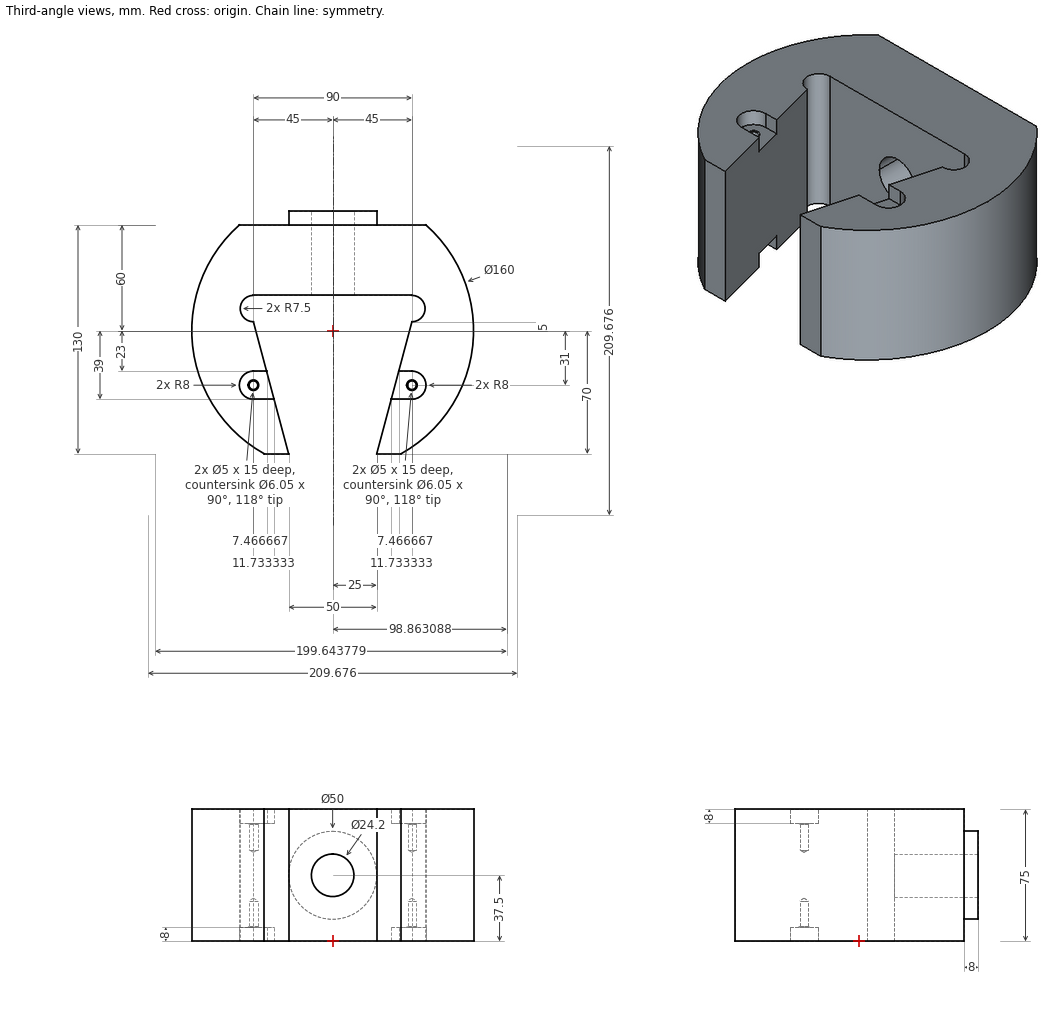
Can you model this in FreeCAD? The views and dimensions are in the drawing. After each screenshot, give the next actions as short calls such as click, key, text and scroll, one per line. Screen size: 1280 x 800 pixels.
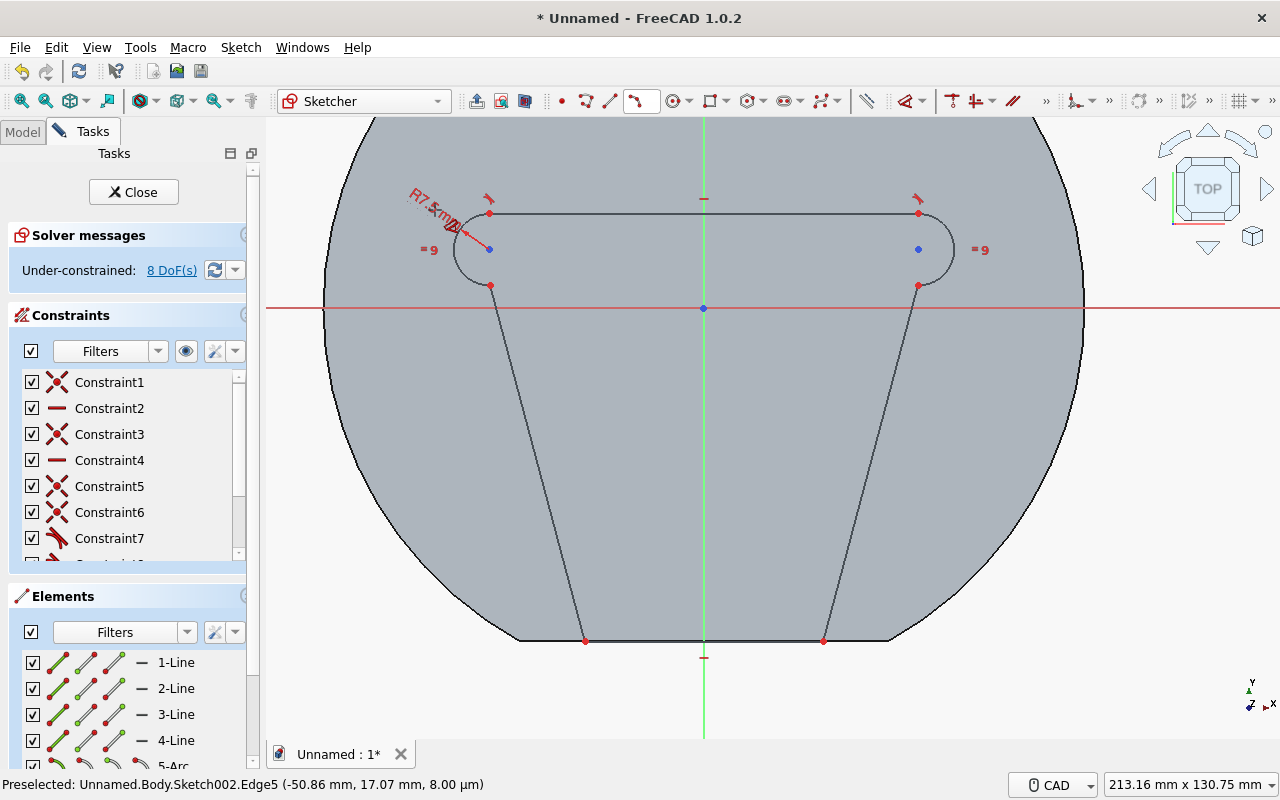
click(752, 642)
click(649, 676)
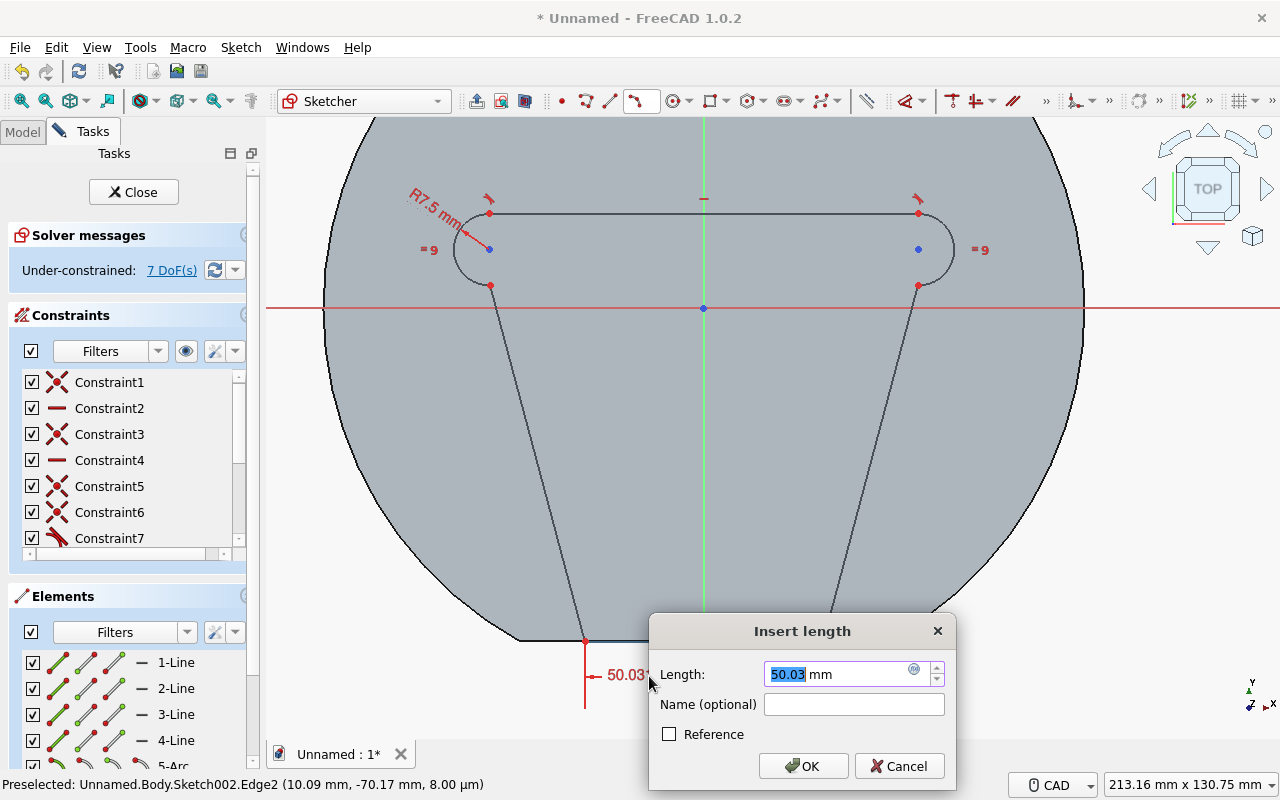
text(50)
key(Return)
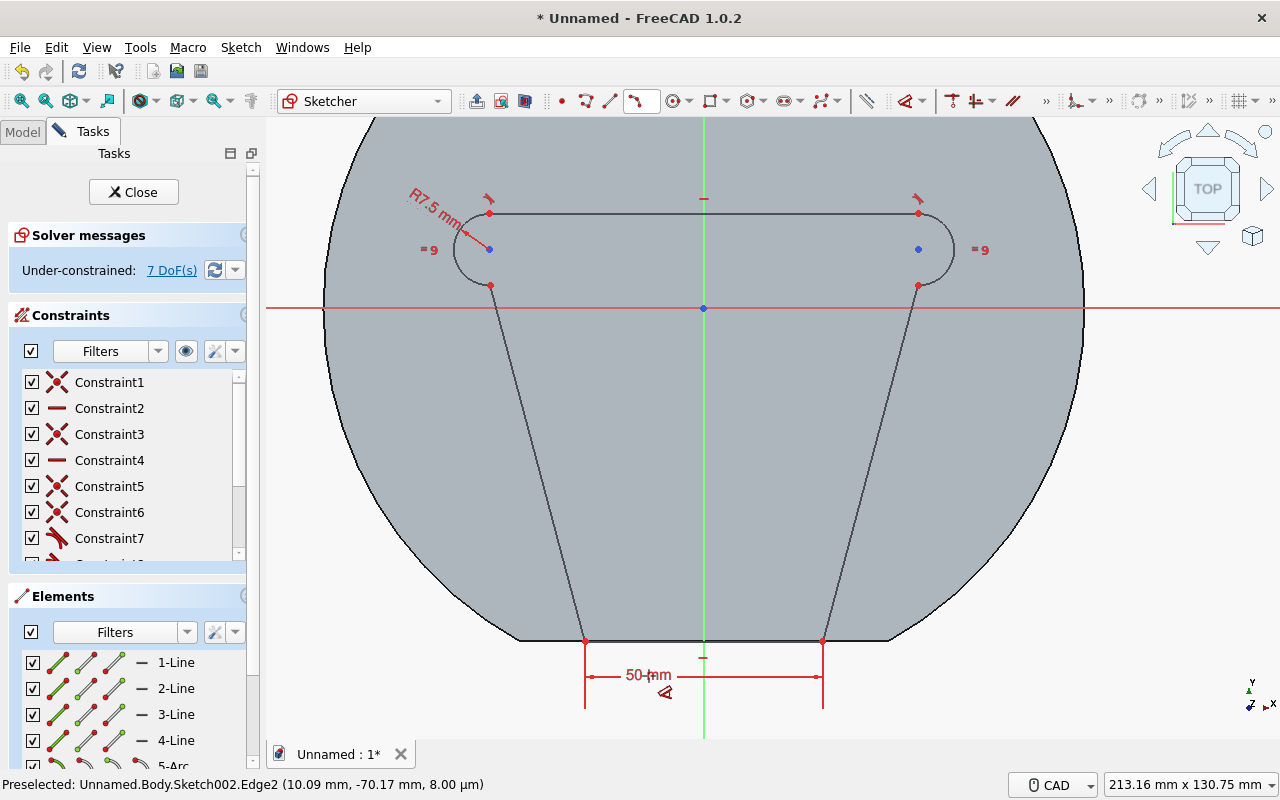
click(618, 214)
click(605, 180)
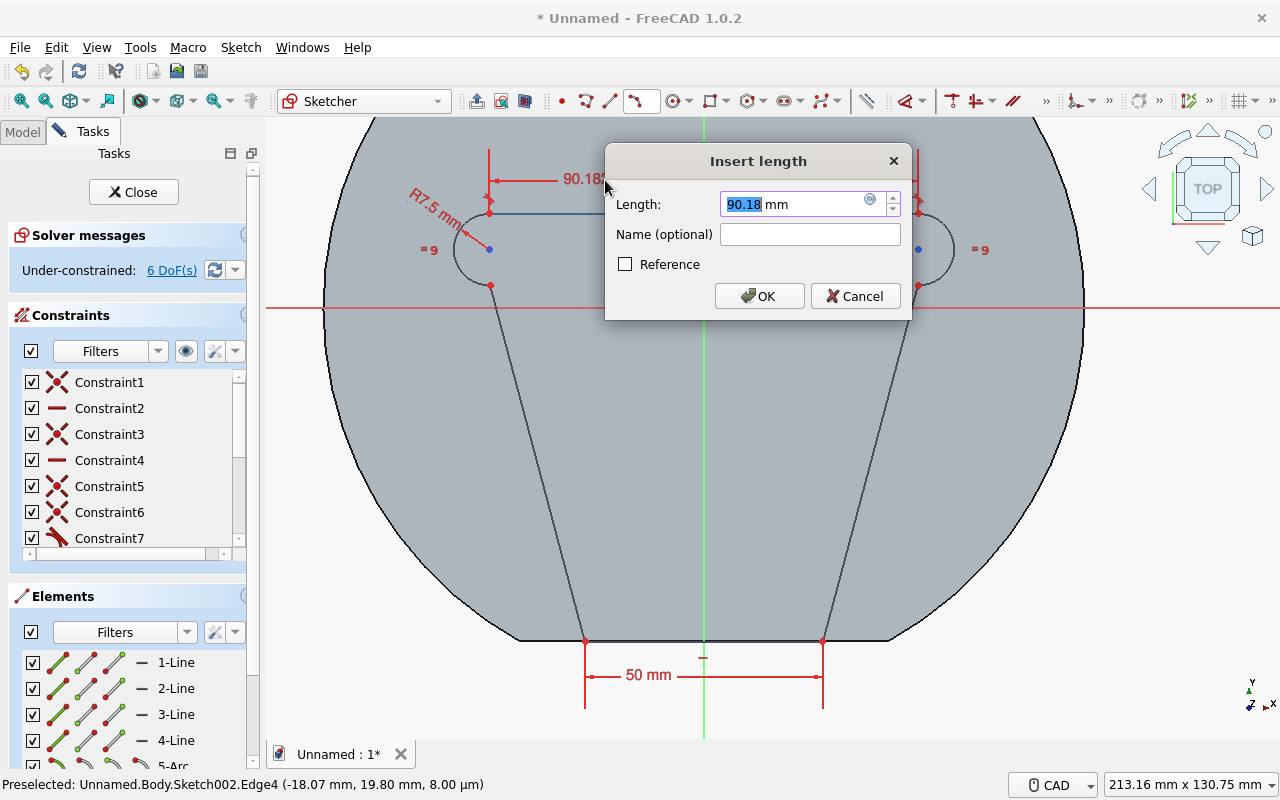
text(90)
key(Return)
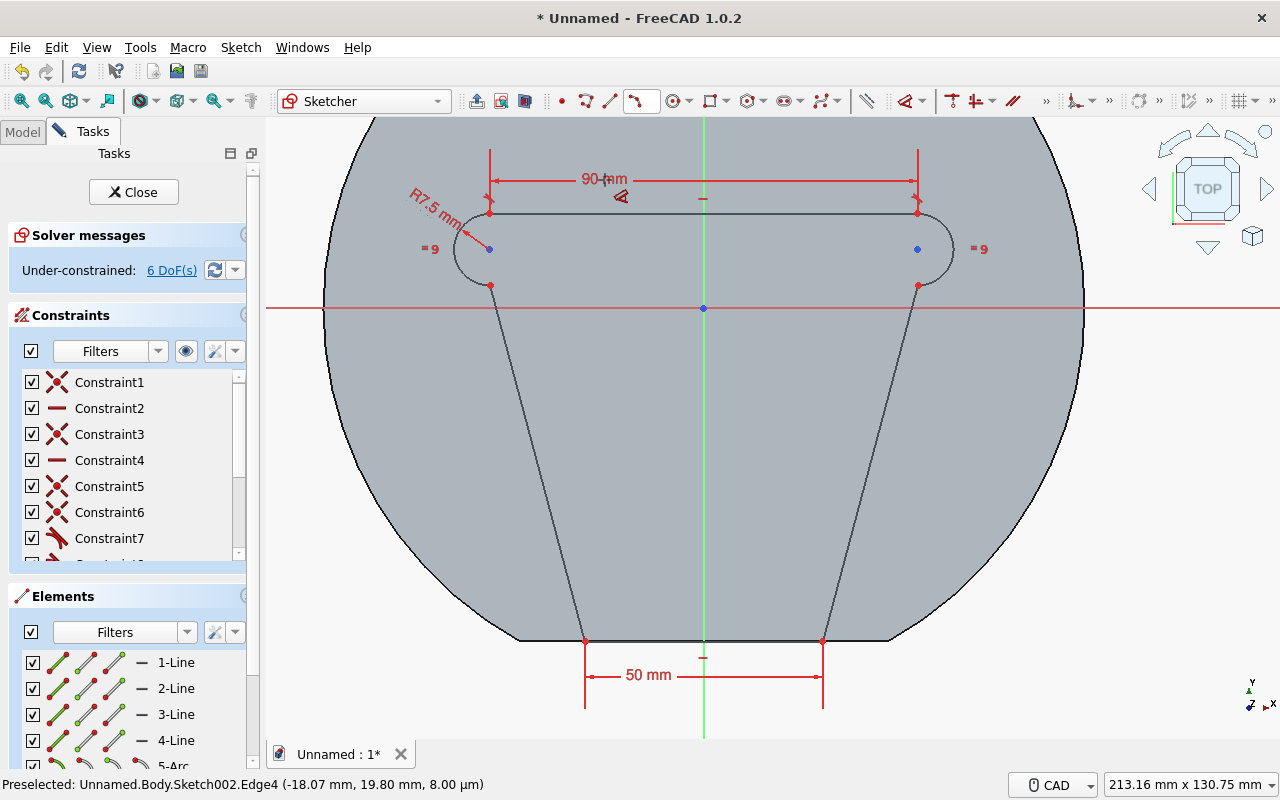
scroll(918, 285, up, 3)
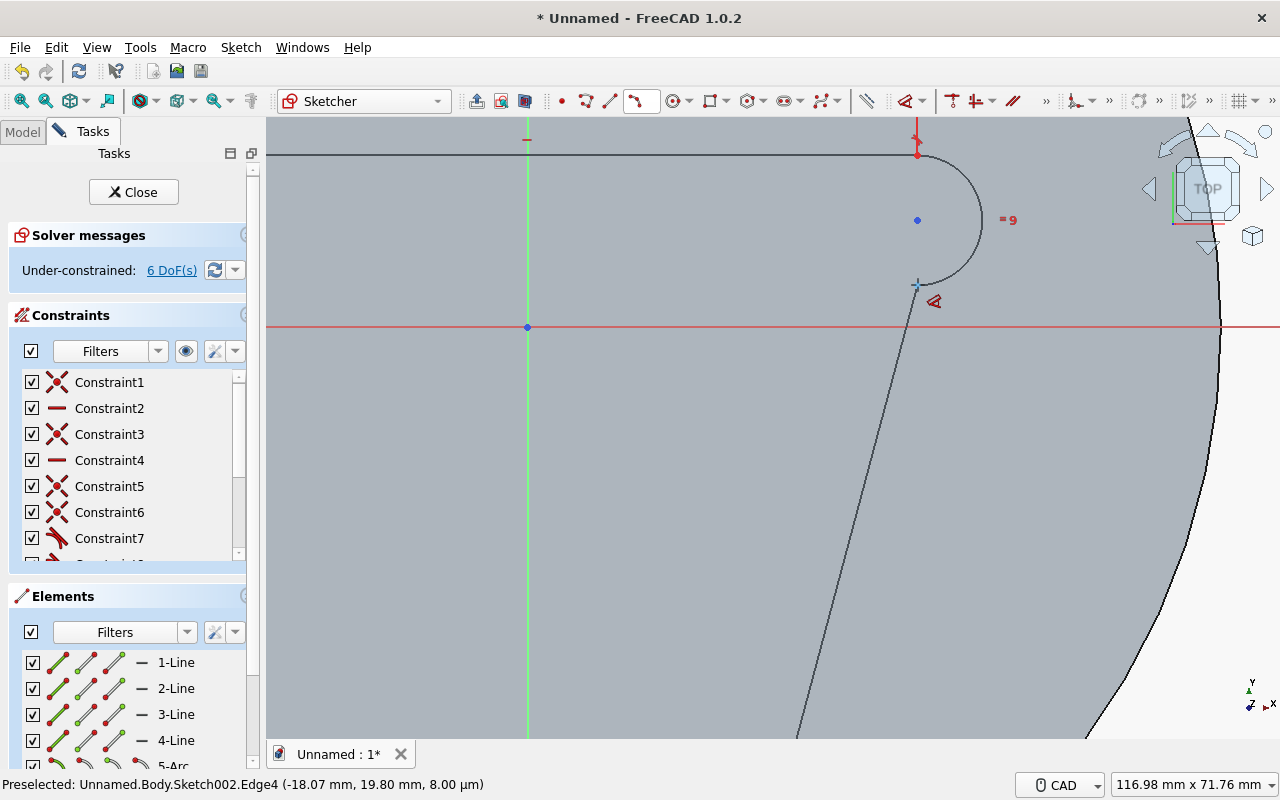
click(917, 285)
click(951, 306)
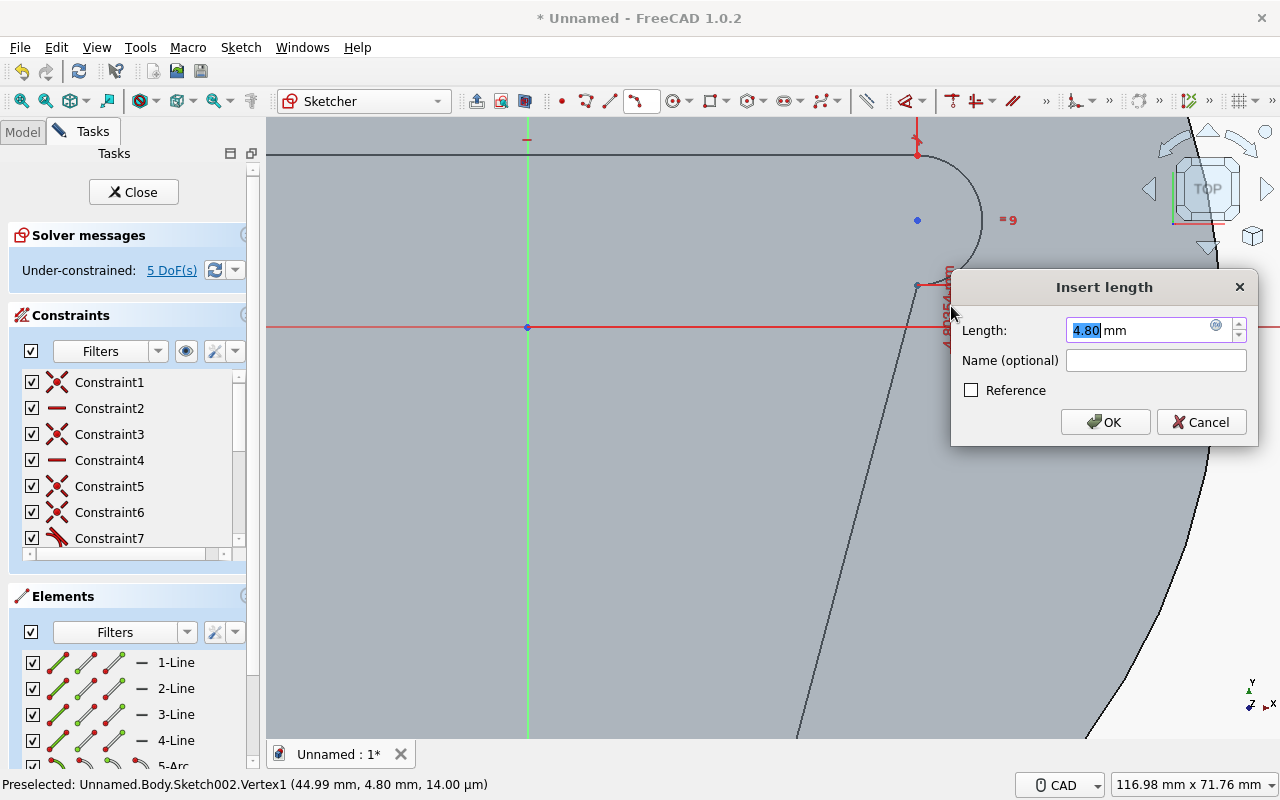
text(5)
key(Return)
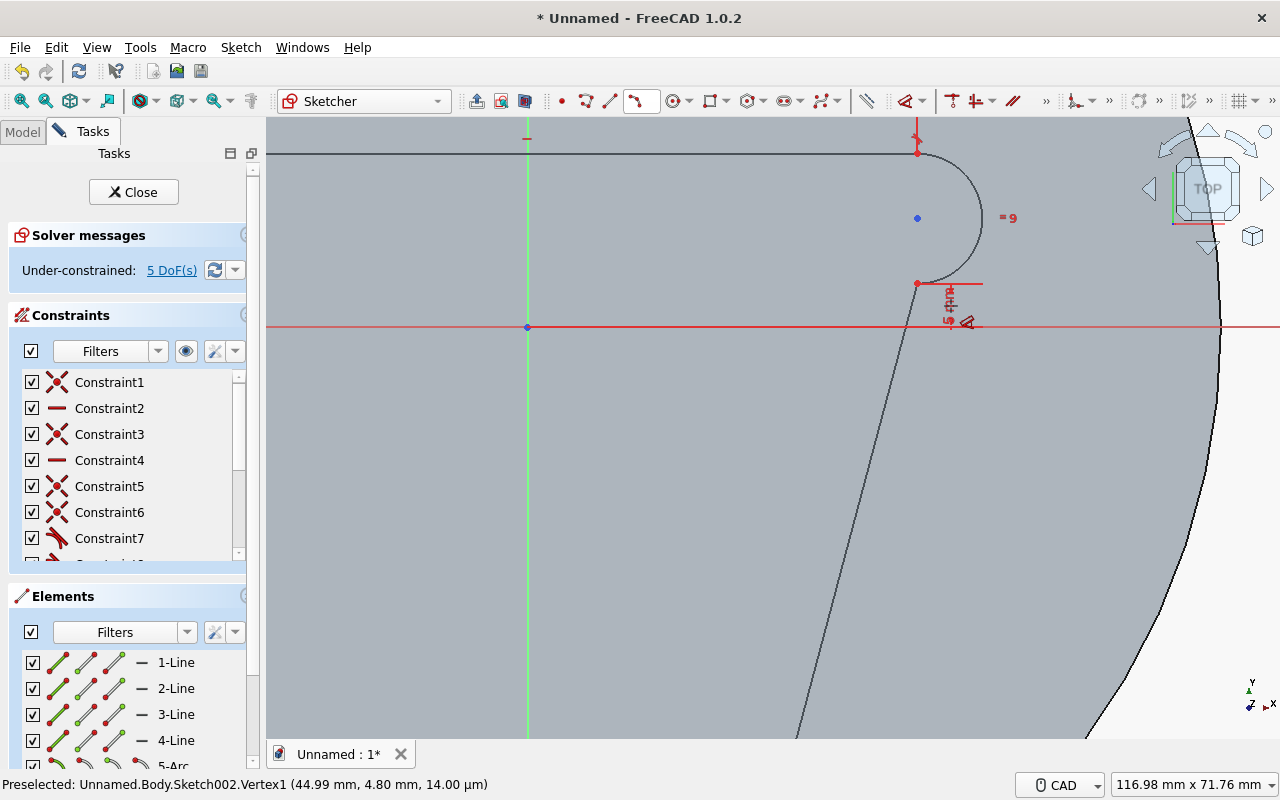
click(917, 284)
click(722, 250)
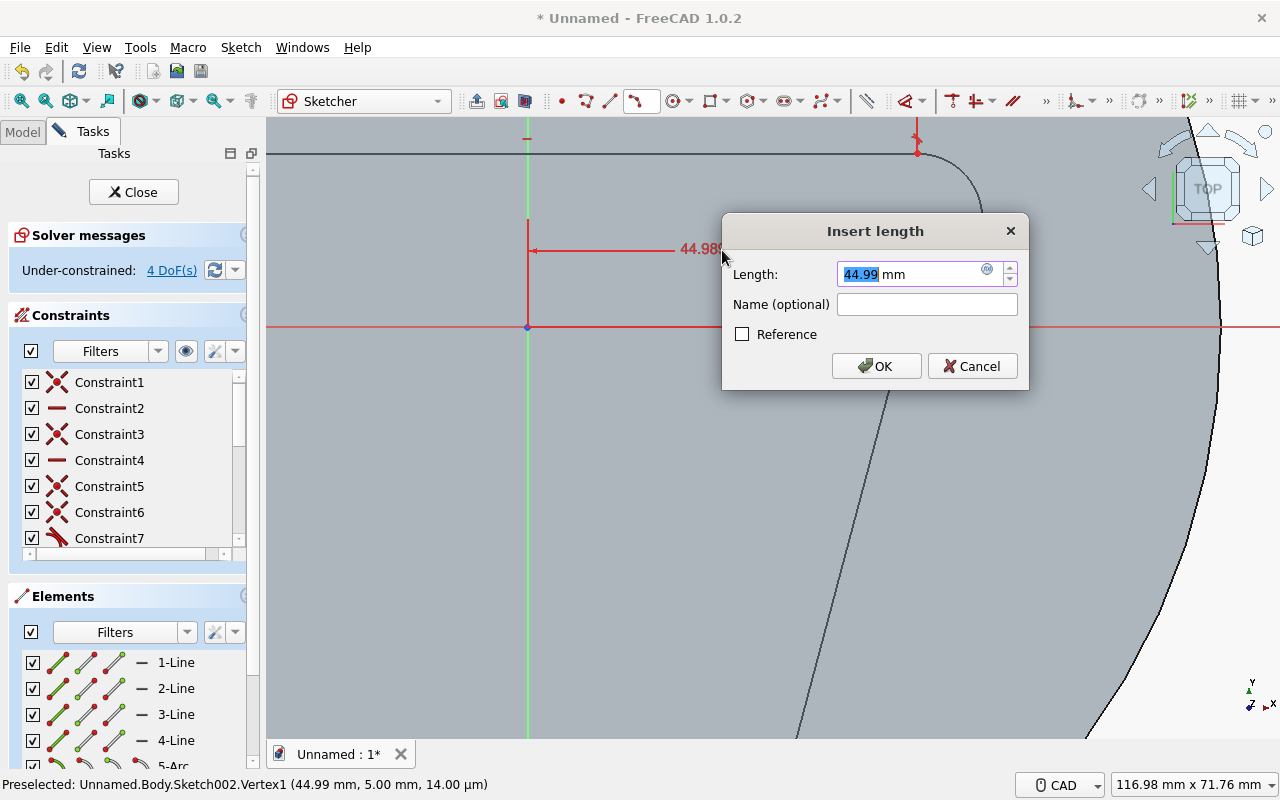
text(45)
key(Return)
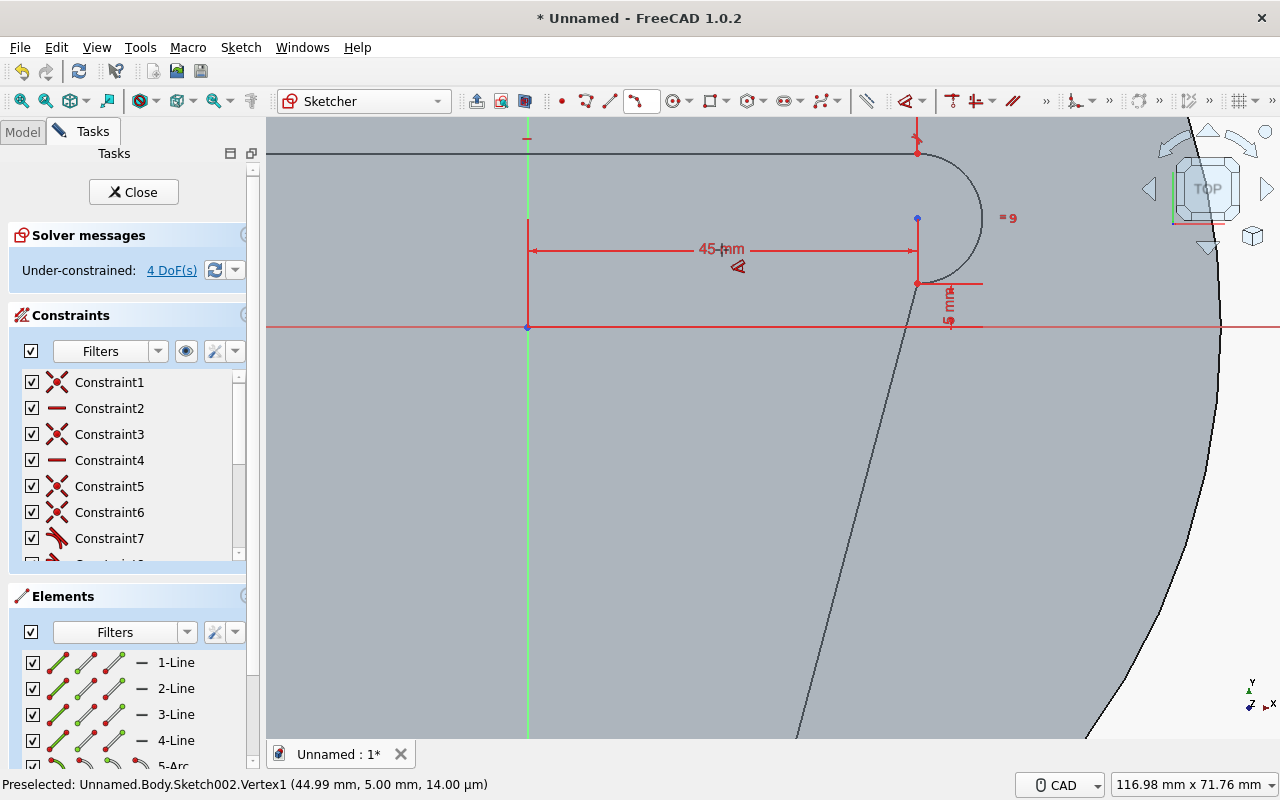
scroll(920, 287, down, 3)